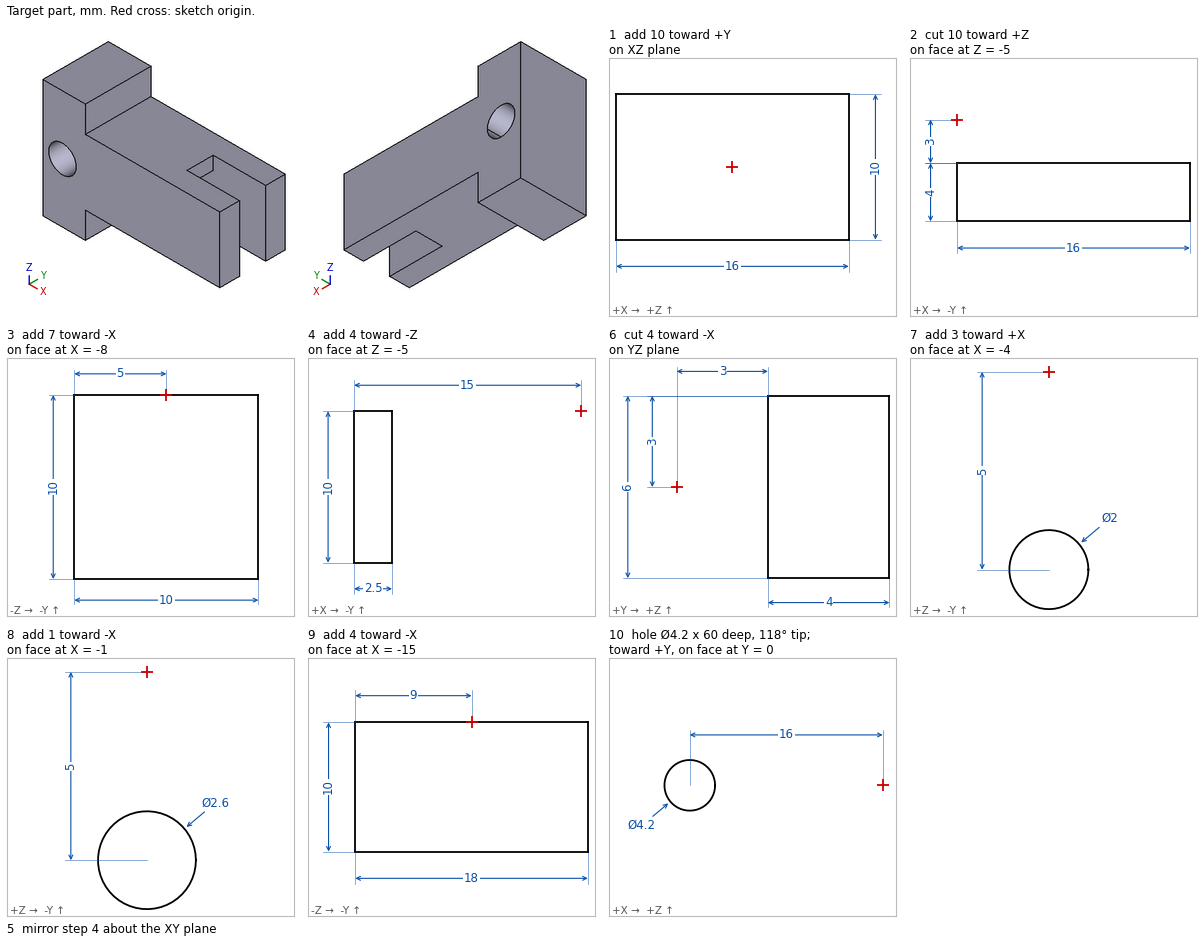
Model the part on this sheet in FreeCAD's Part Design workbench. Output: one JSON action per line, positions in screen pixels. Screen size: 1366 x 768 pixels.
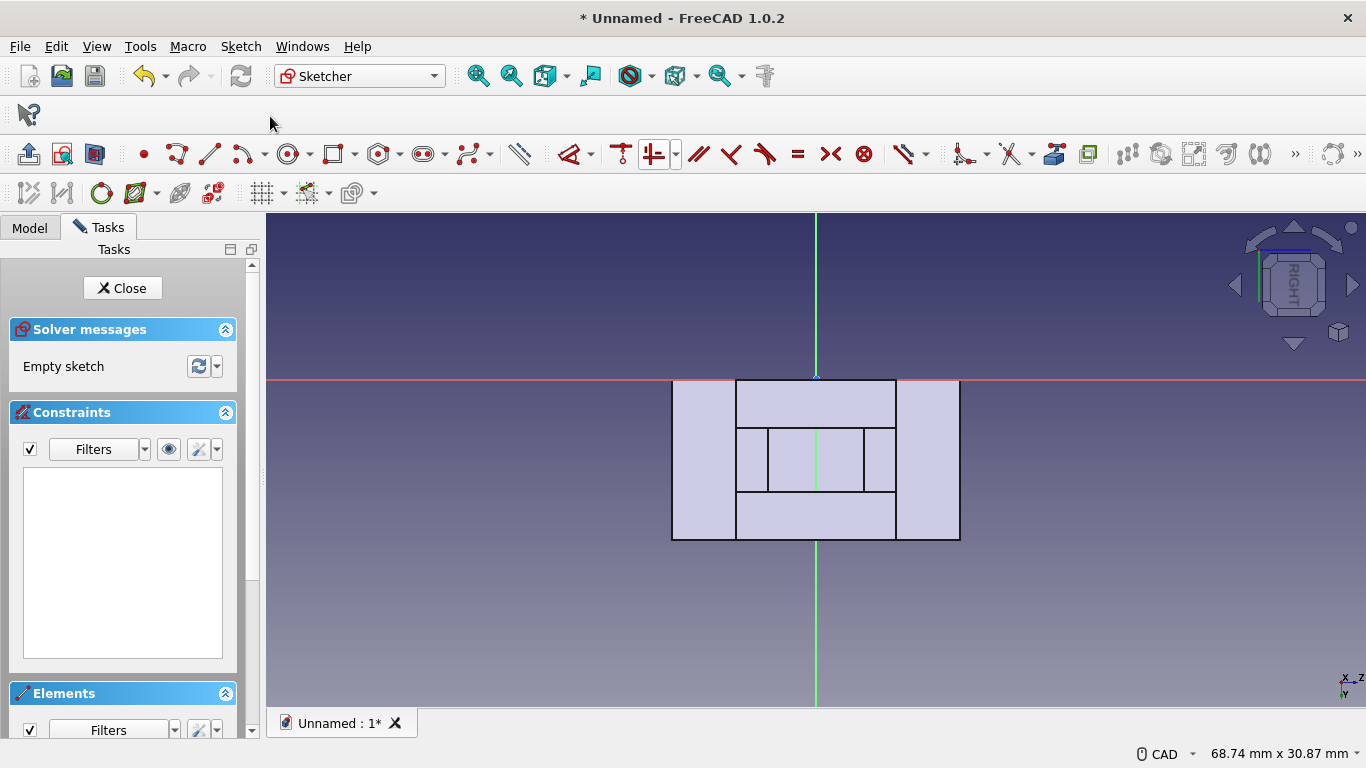
{"action": "left_click", "coordinate": [95, 154]}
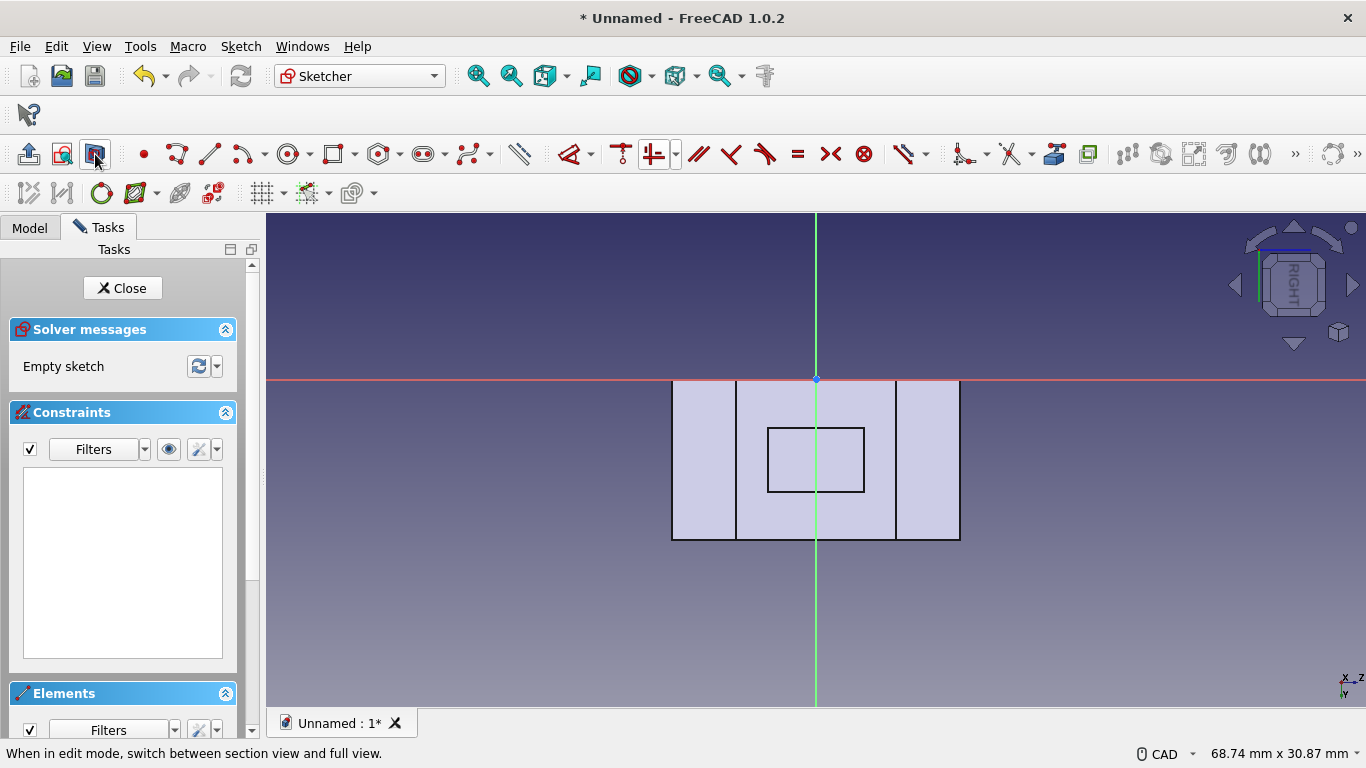
{"action": "scroll", "coordinate": [825, 460], "scroll_direction": "up", "scroll_amount": 11}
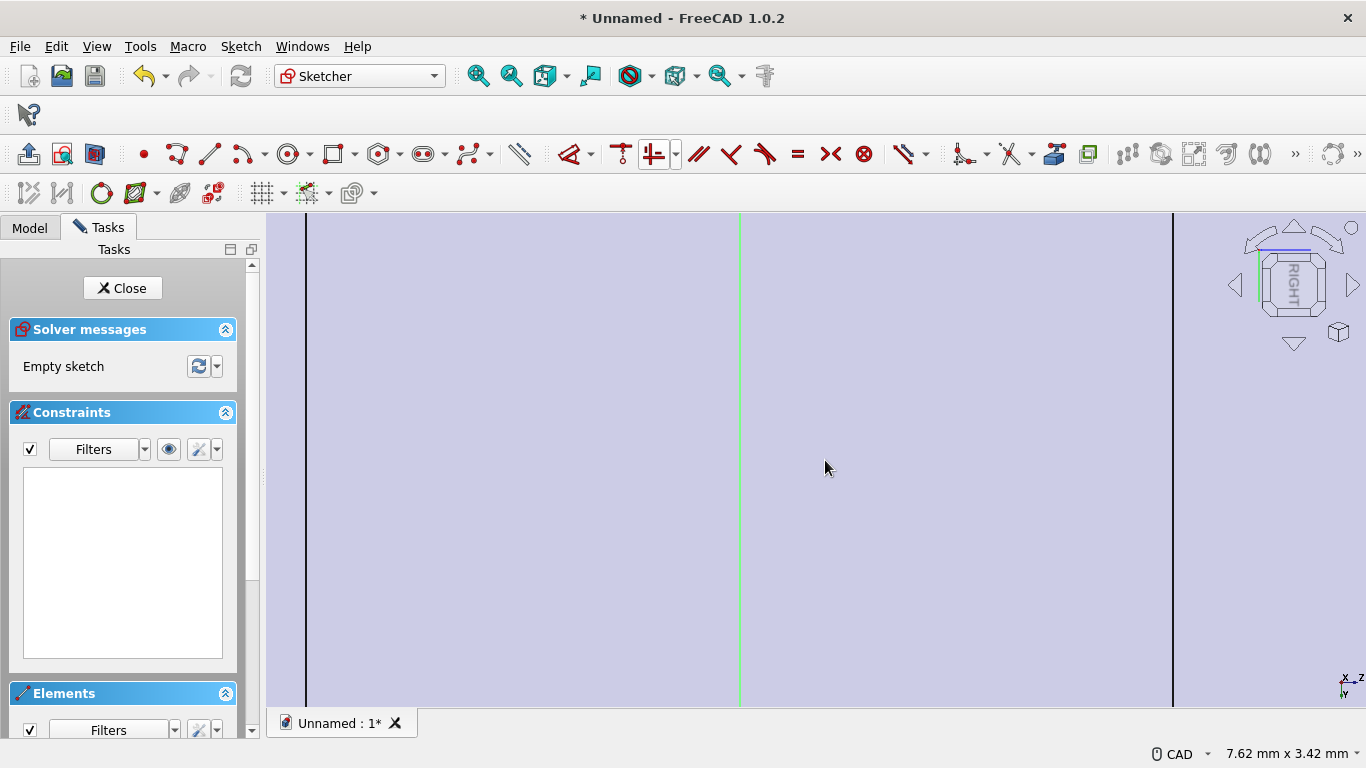
{"action": "left_click", "coordinate": [288, 154]}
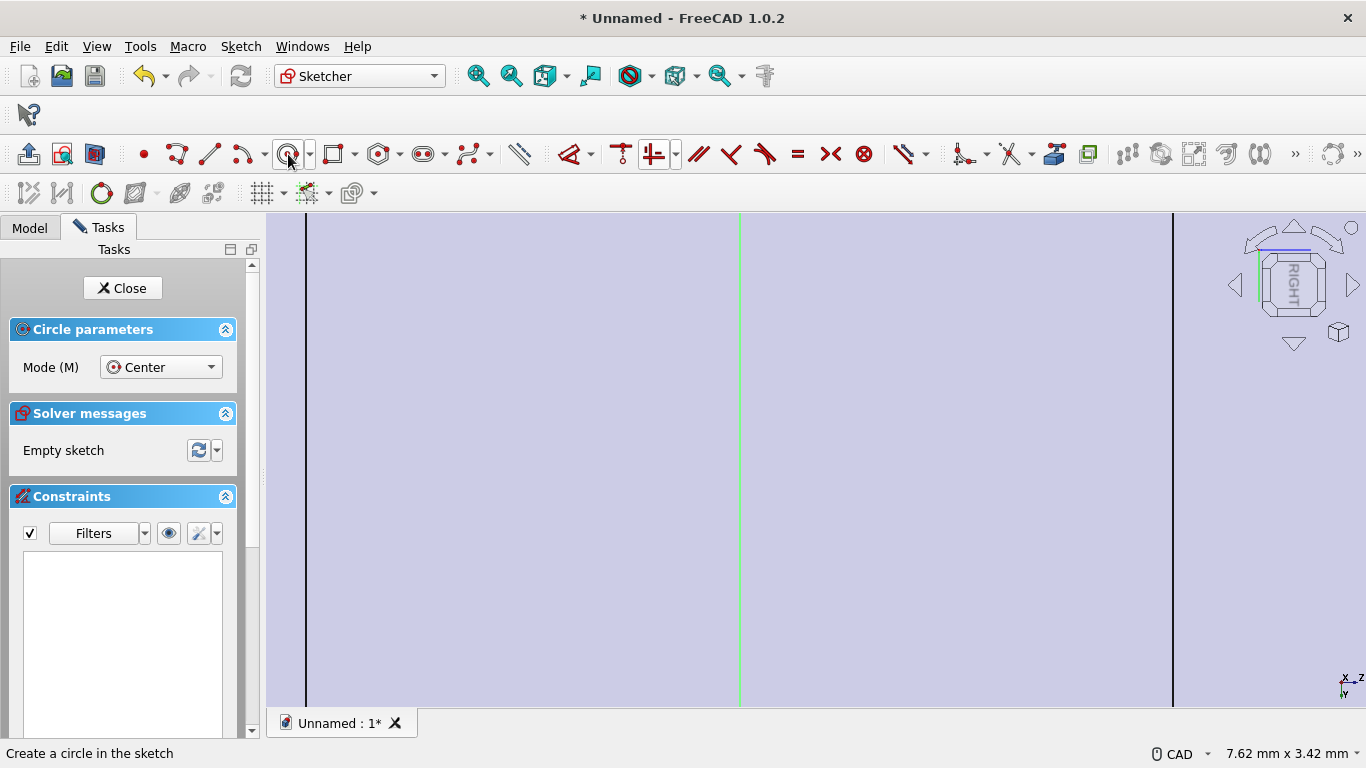
{"action": "left_click", "coordinate": [740, 456]}
{"action": "left_click", "coordinate": [842, 354]}
{"action": "key", "text": "Escape"}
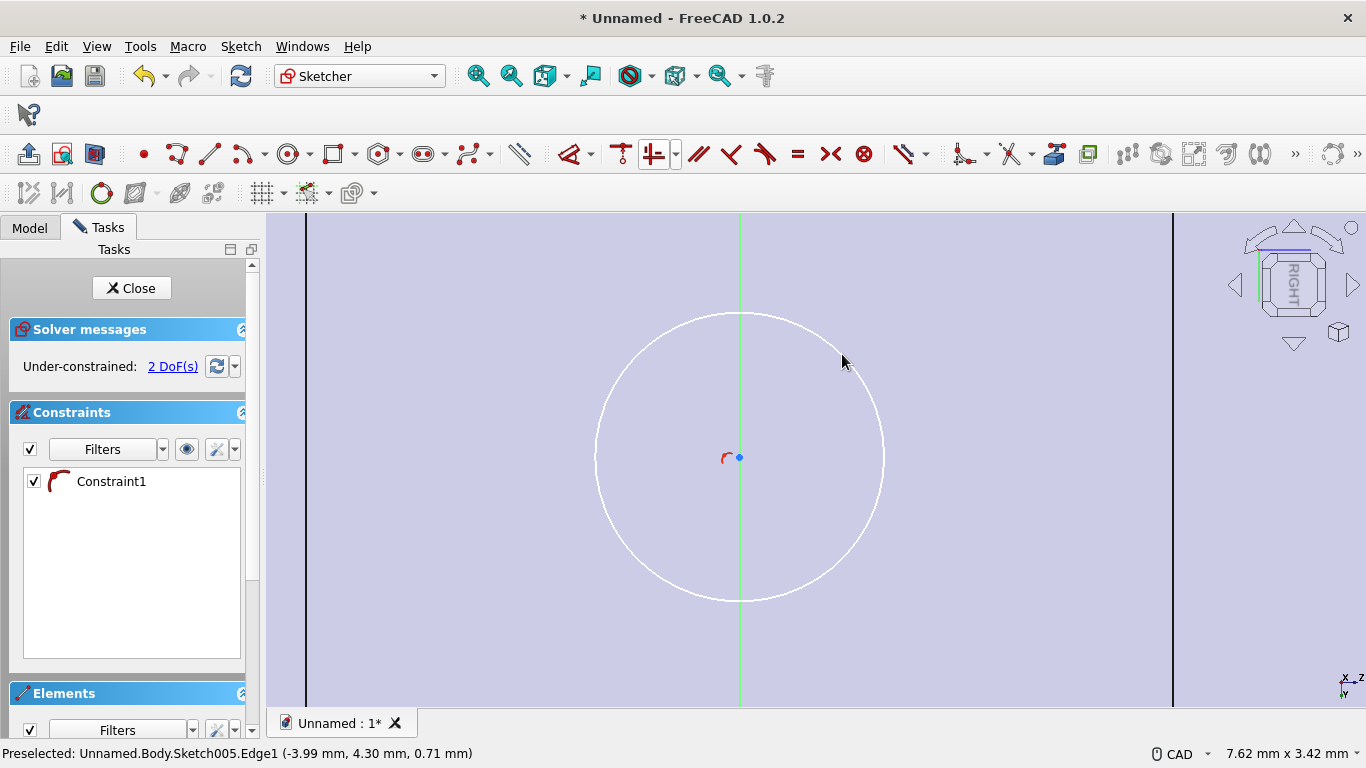
{"action": "left_click", "coordinate": [568, 154]}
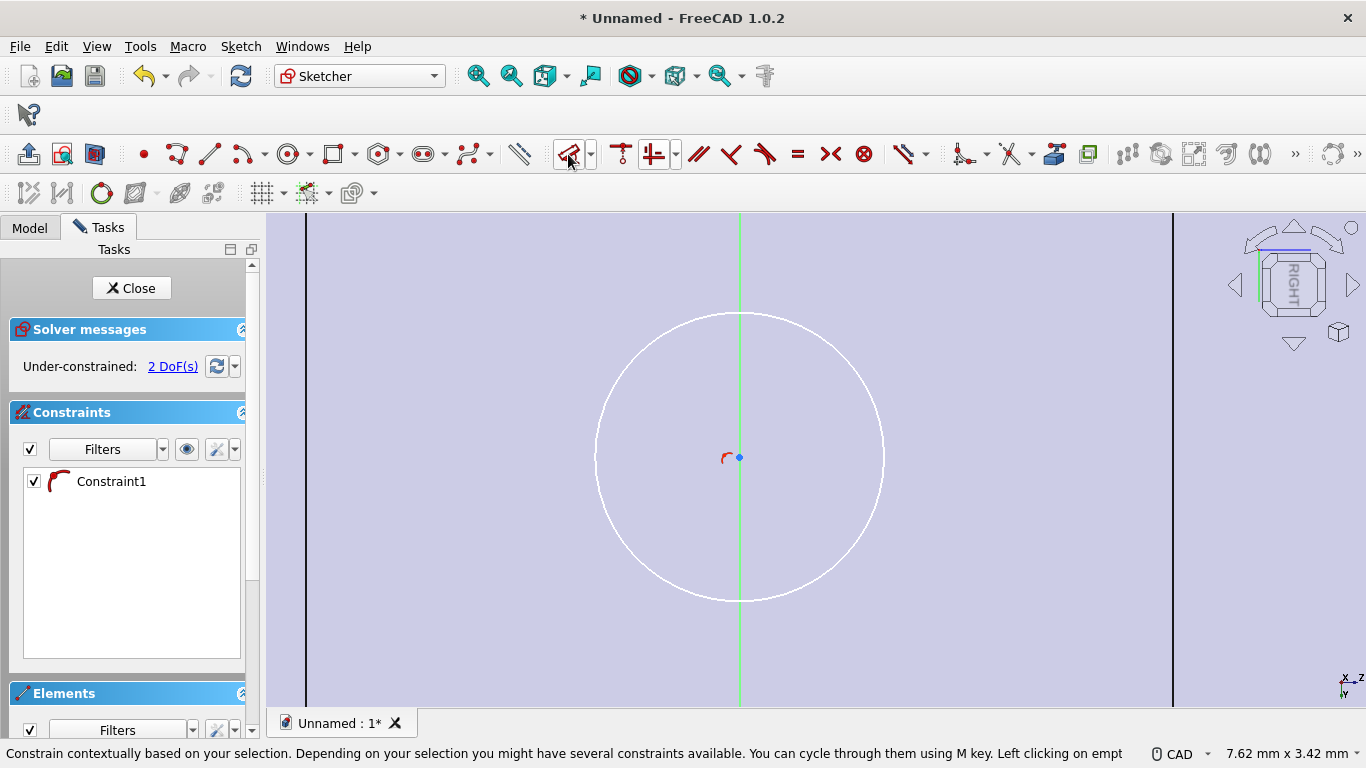
{"action": "left_click", "coordinate": [842, 355]}
{"action": "left_click", "coordinate": [865, 332]}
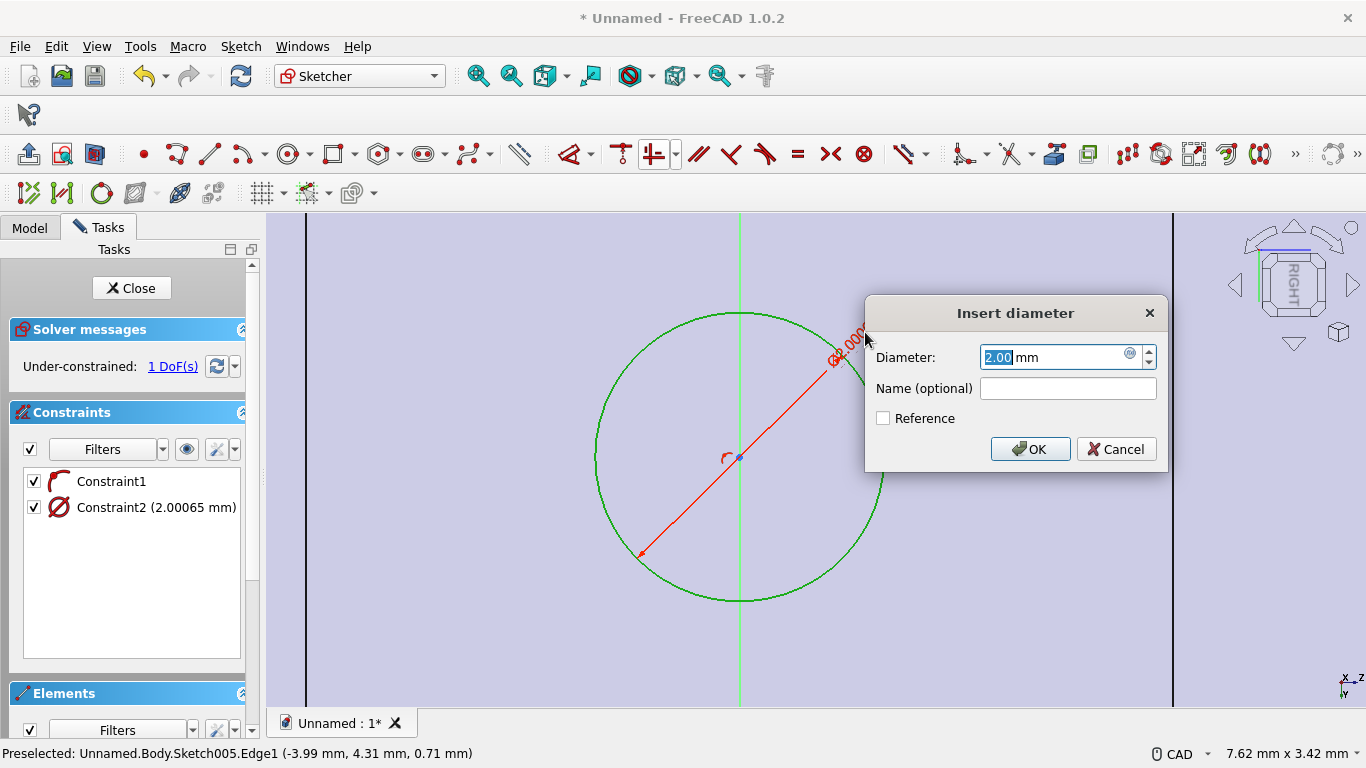
{"action": "type", "text": "2"}
{"action": "key", "text": "Return"}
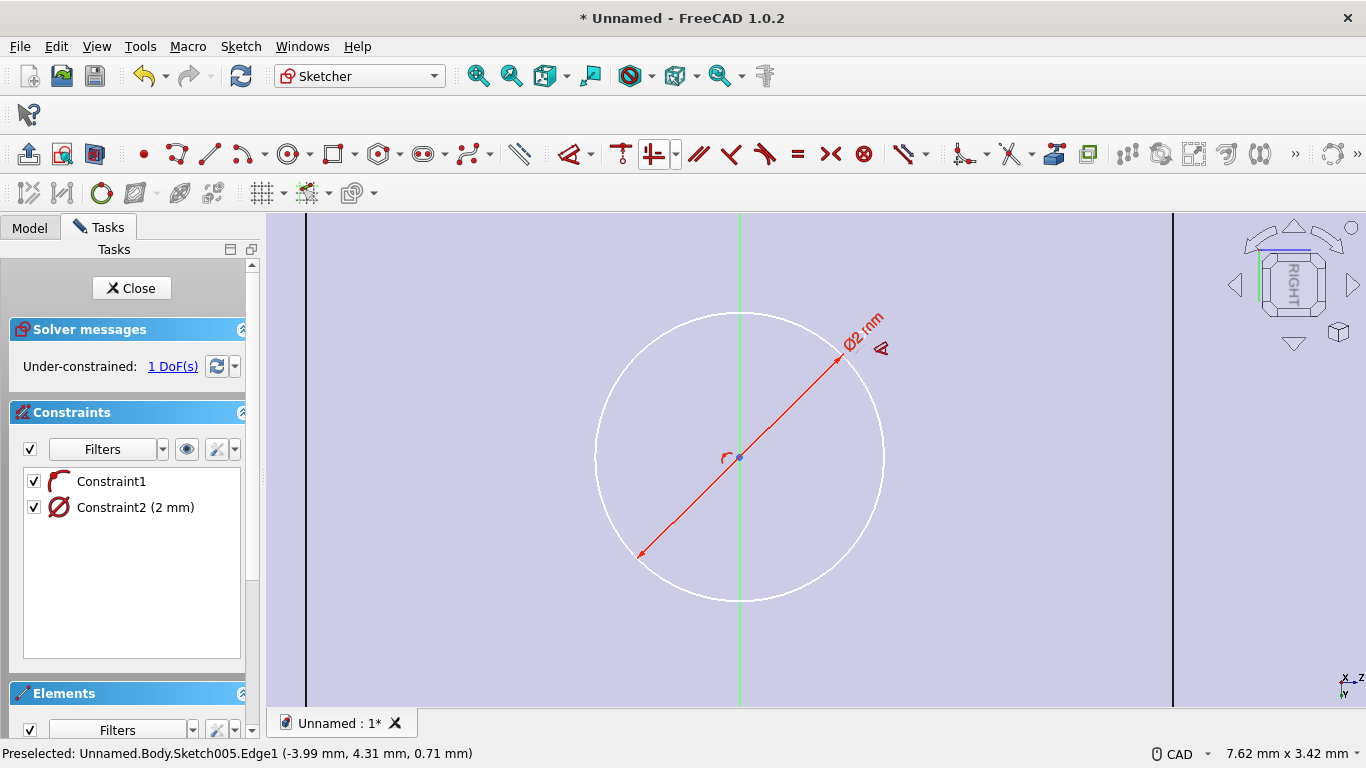
{"action": "left_click", "coordinate": [740, 457]}
{"action": "left_click", "coordinate": [774, 349]}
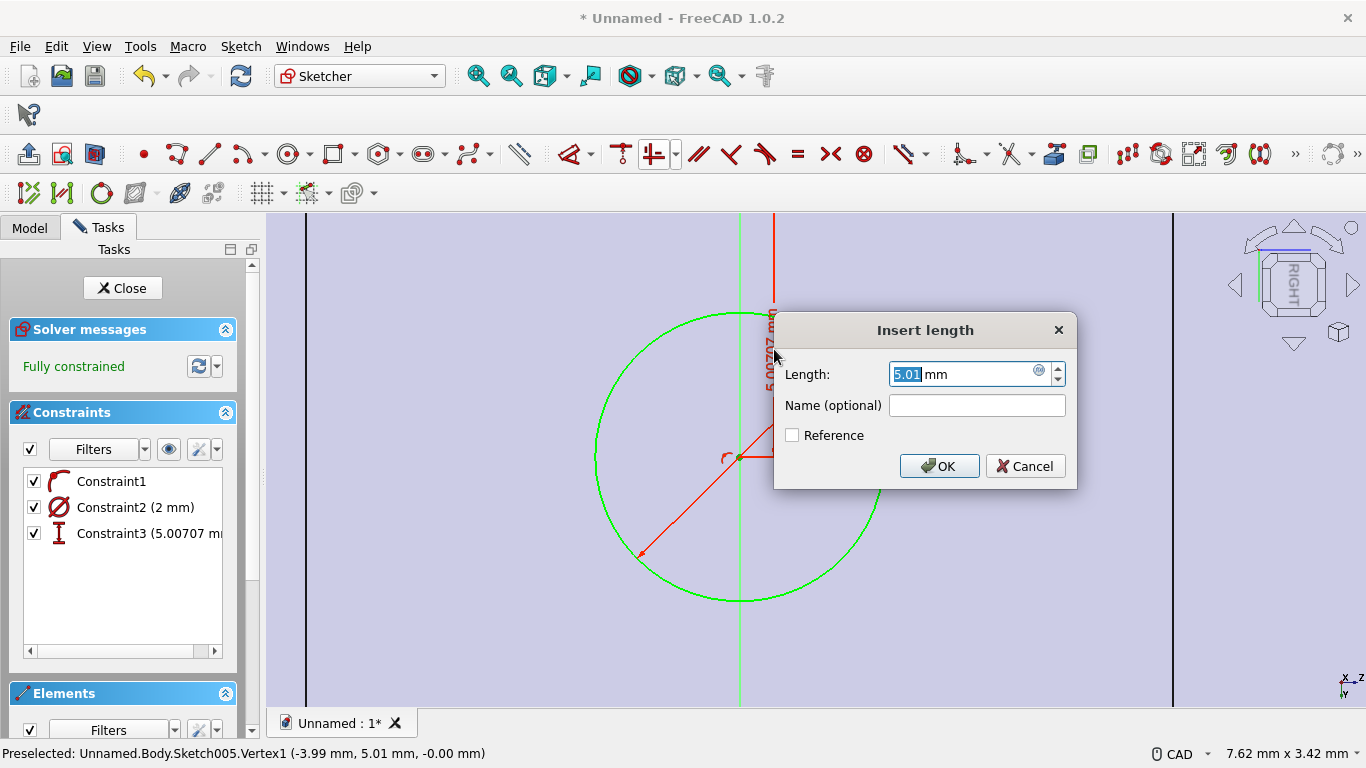
{"action": "type", "text": "5"}
{"action": "key", "text": "Return"}
{"action": "key", "text": "Escape"}